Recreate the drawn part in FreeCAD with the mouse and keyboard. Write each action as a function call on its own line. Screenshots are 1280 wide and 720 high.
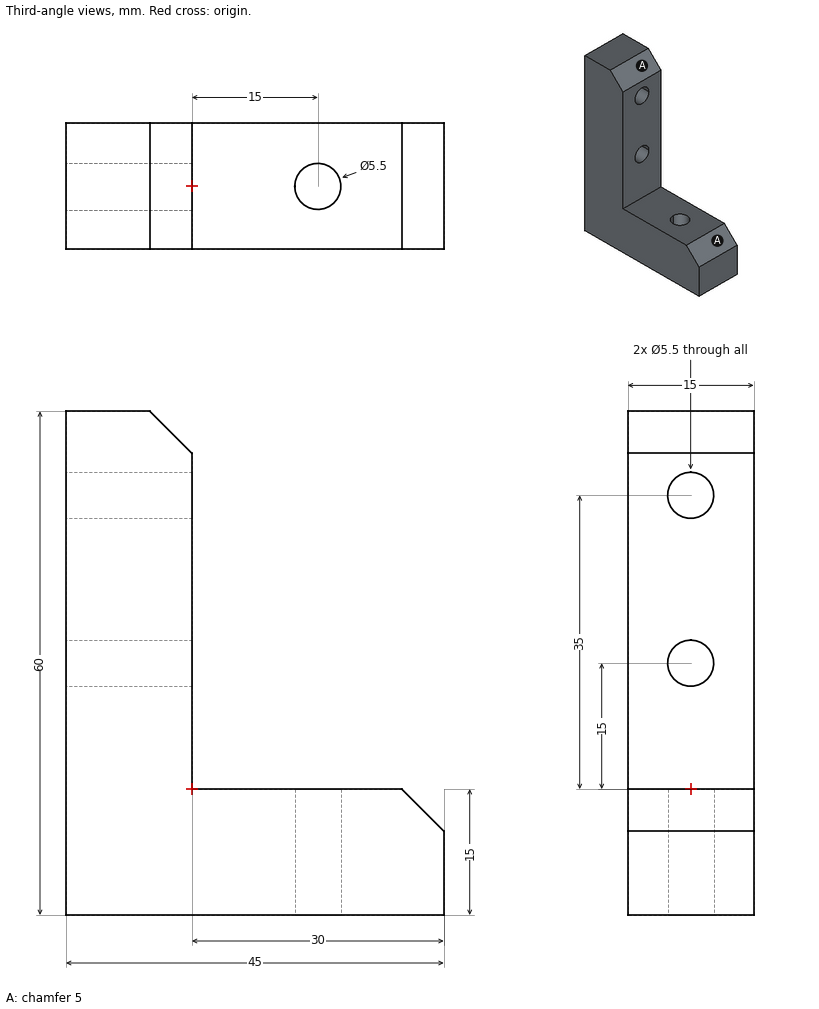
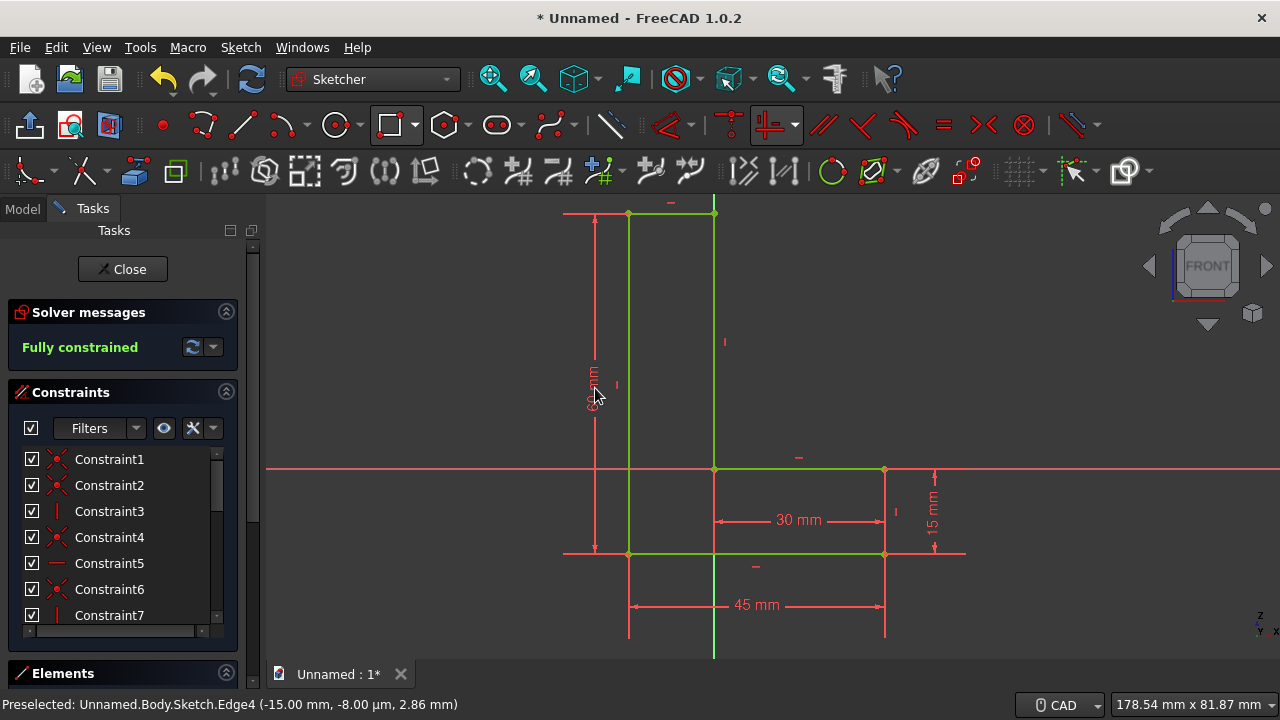
click(123, 269)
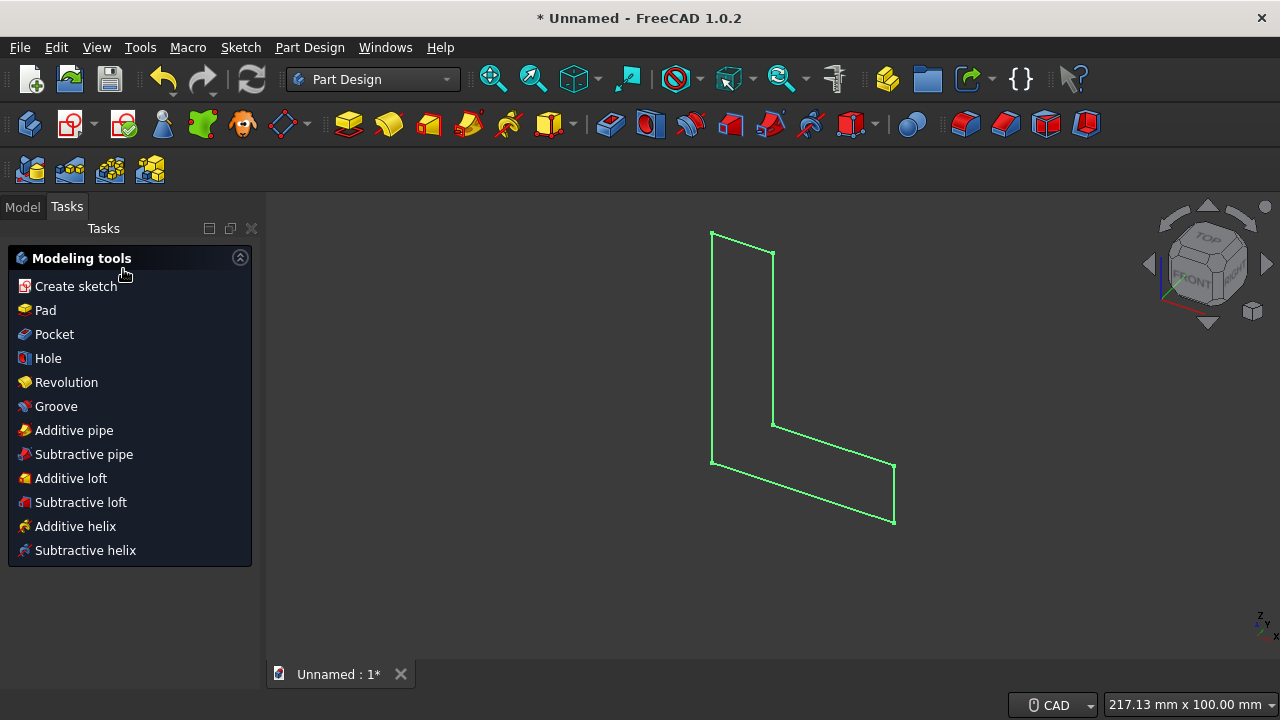
click(350, 124)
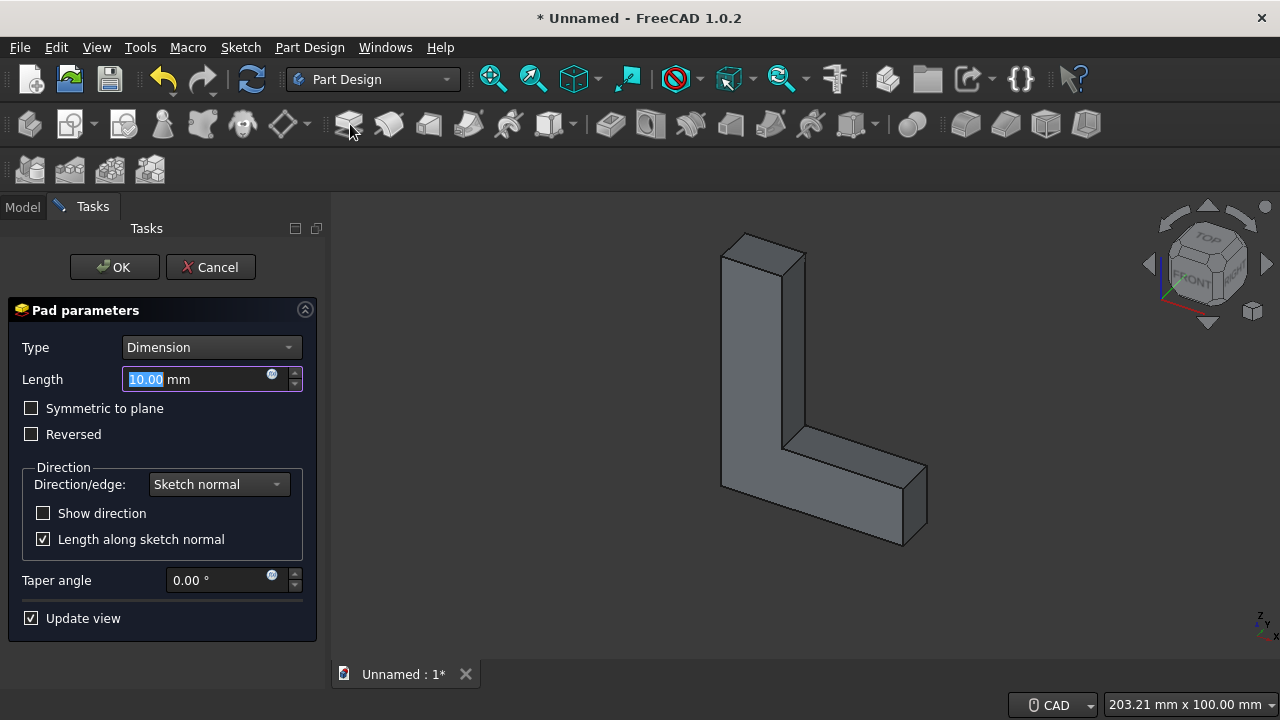
text(15)
key(Tab)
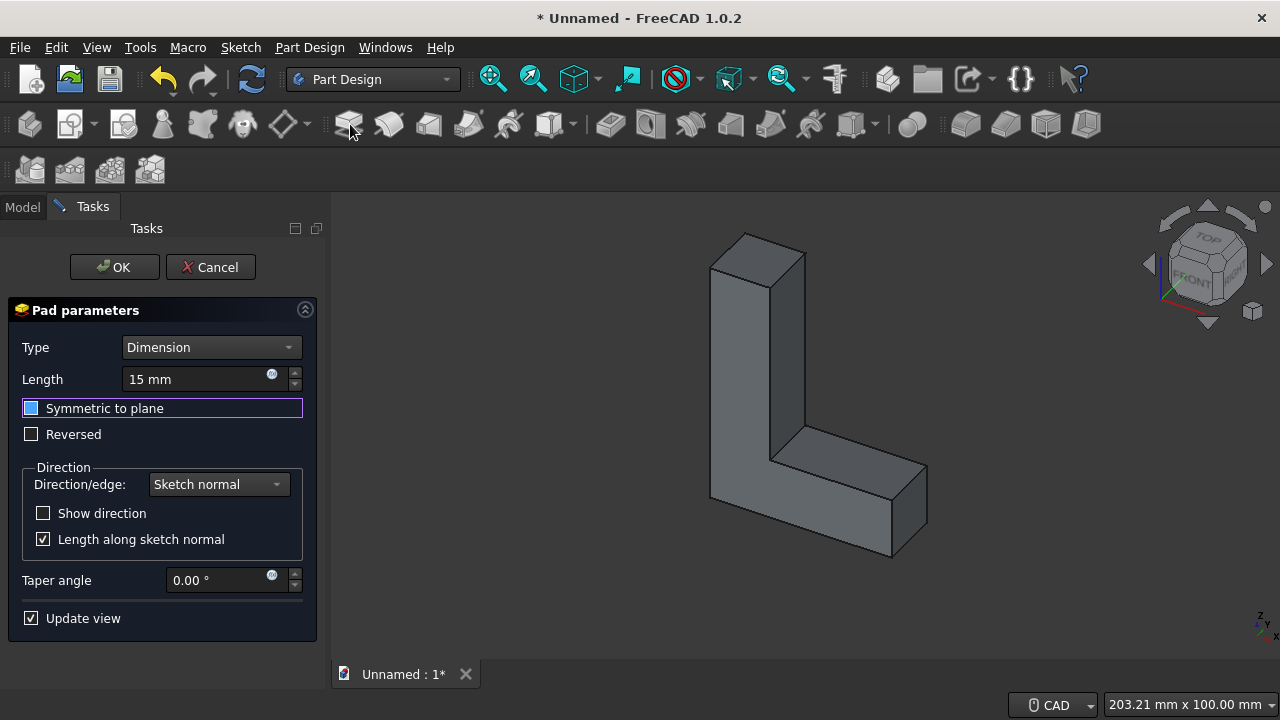
click(30, 408)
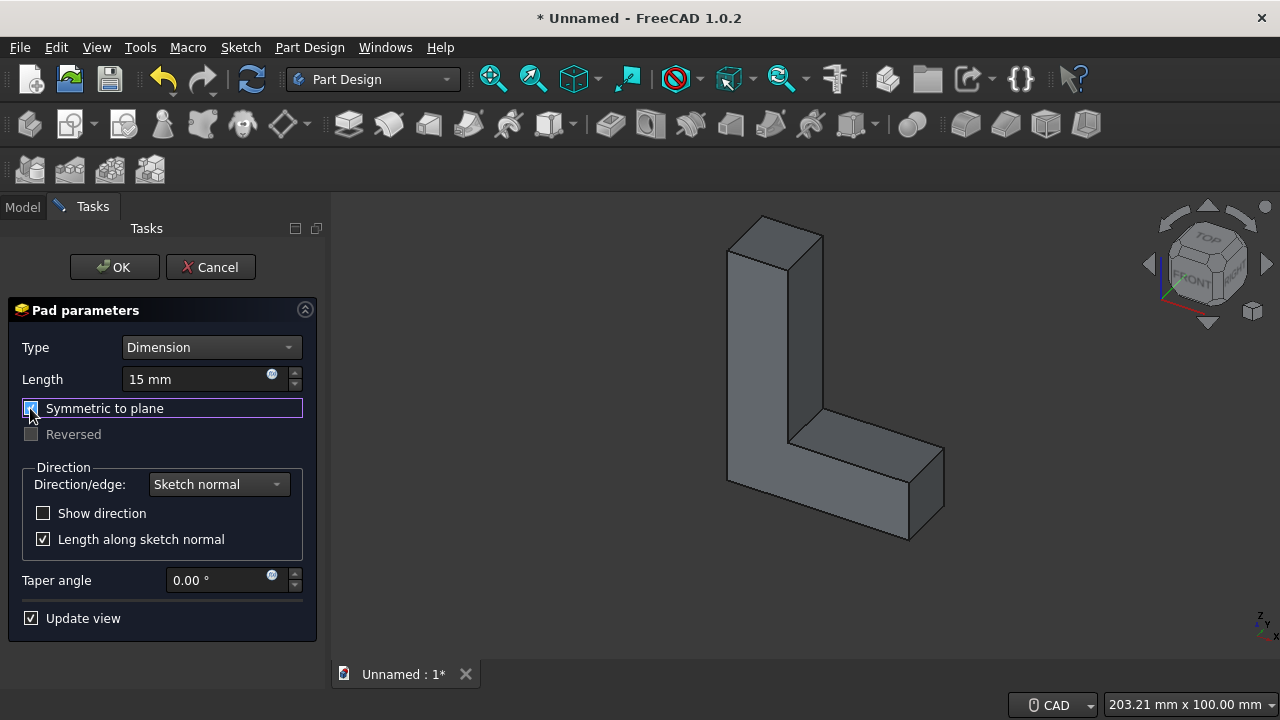
click(115, 267)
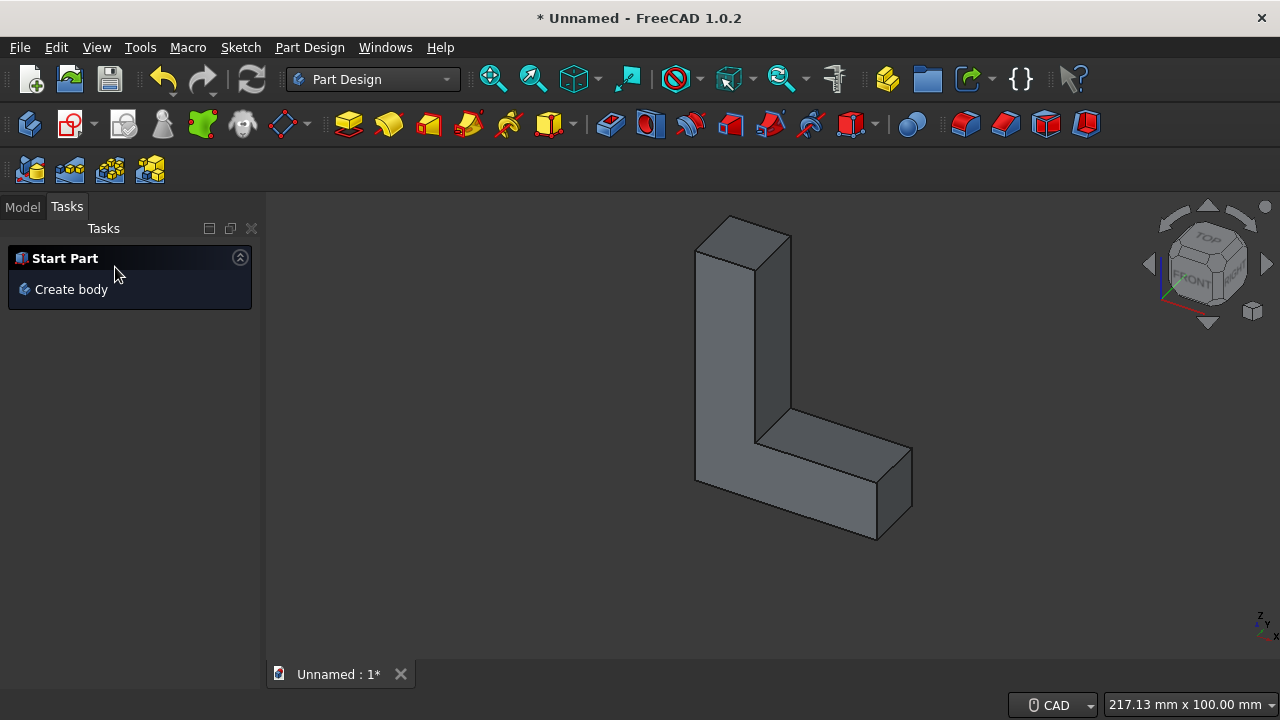
click(894, 465)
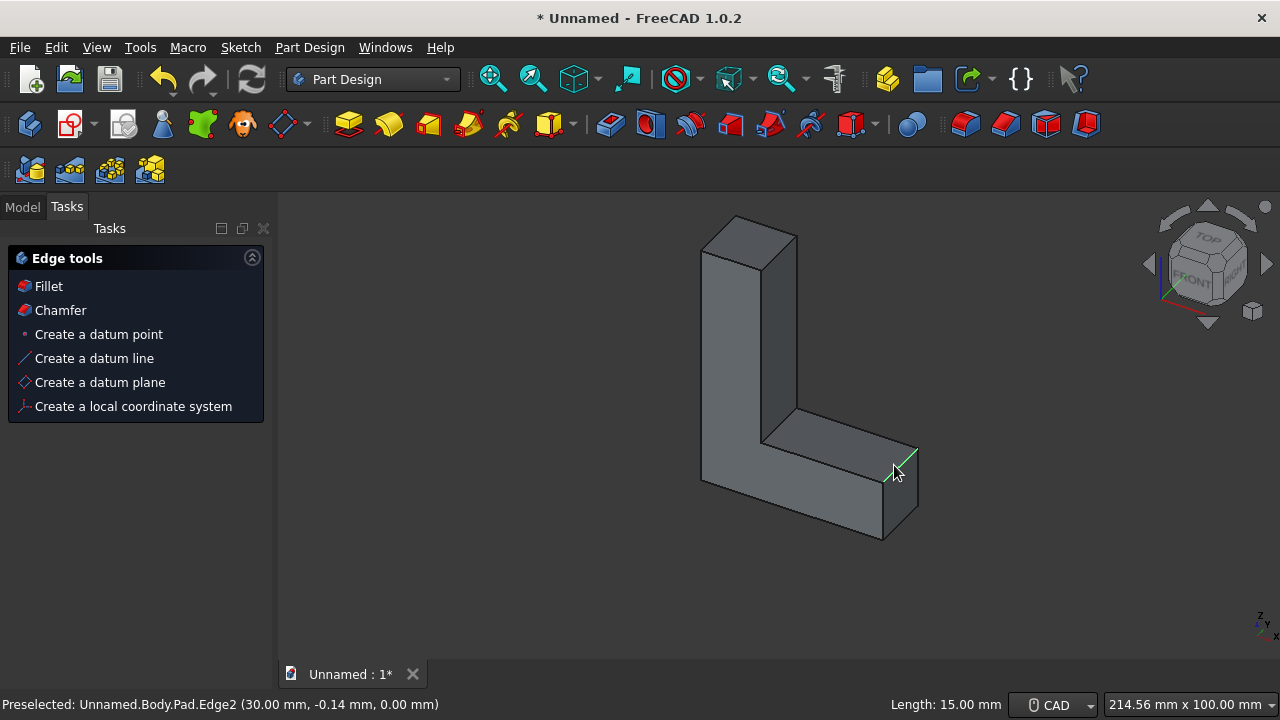
click(779, 252, ctrl)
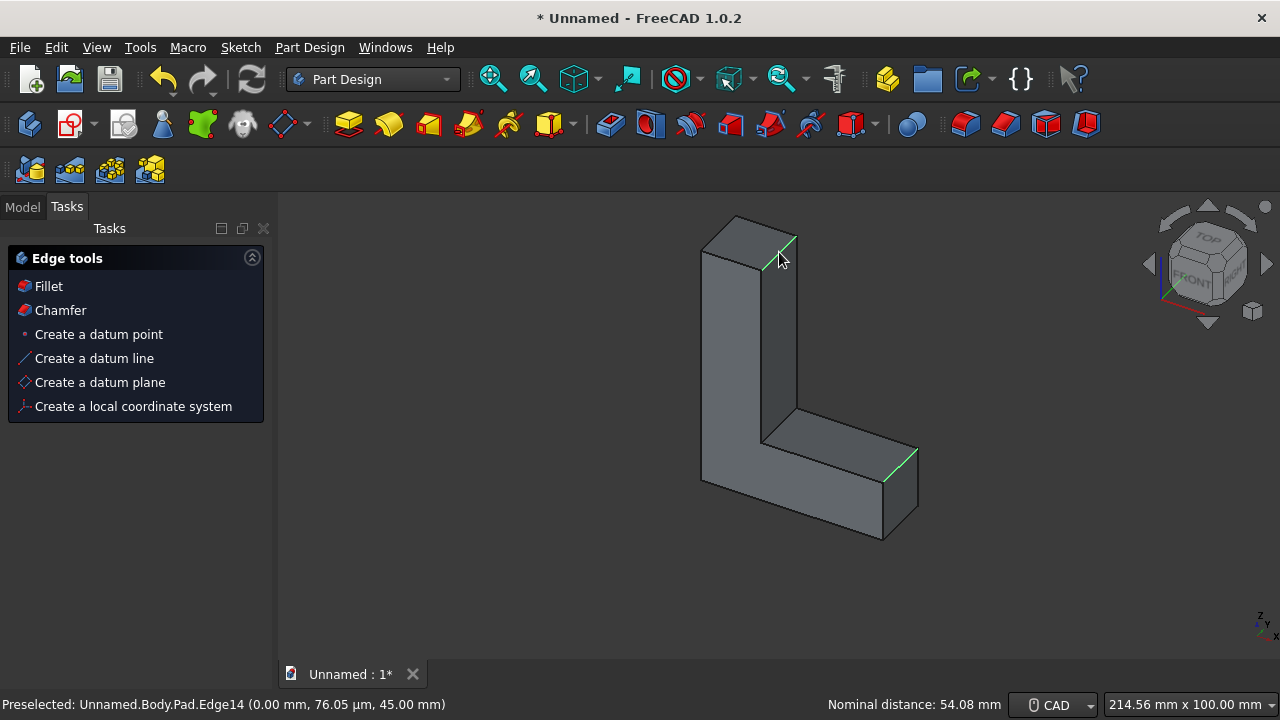
click(1006, 124)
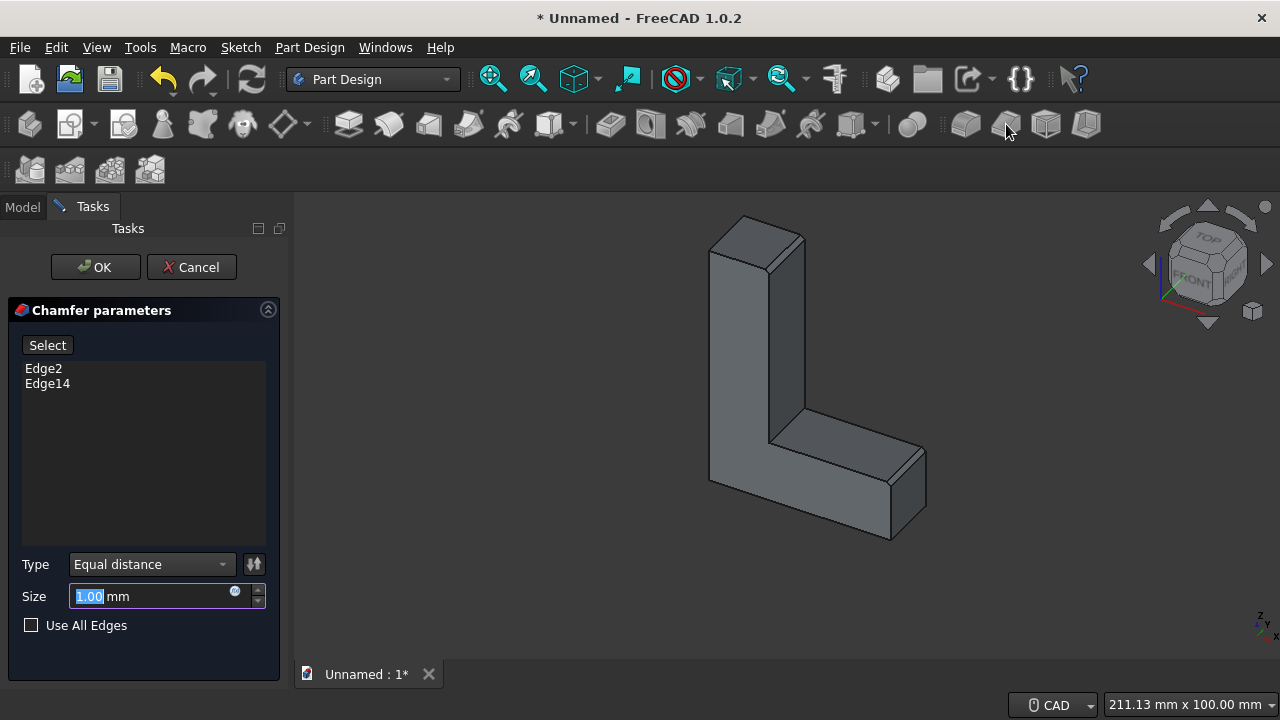
text(5)
key(Tab)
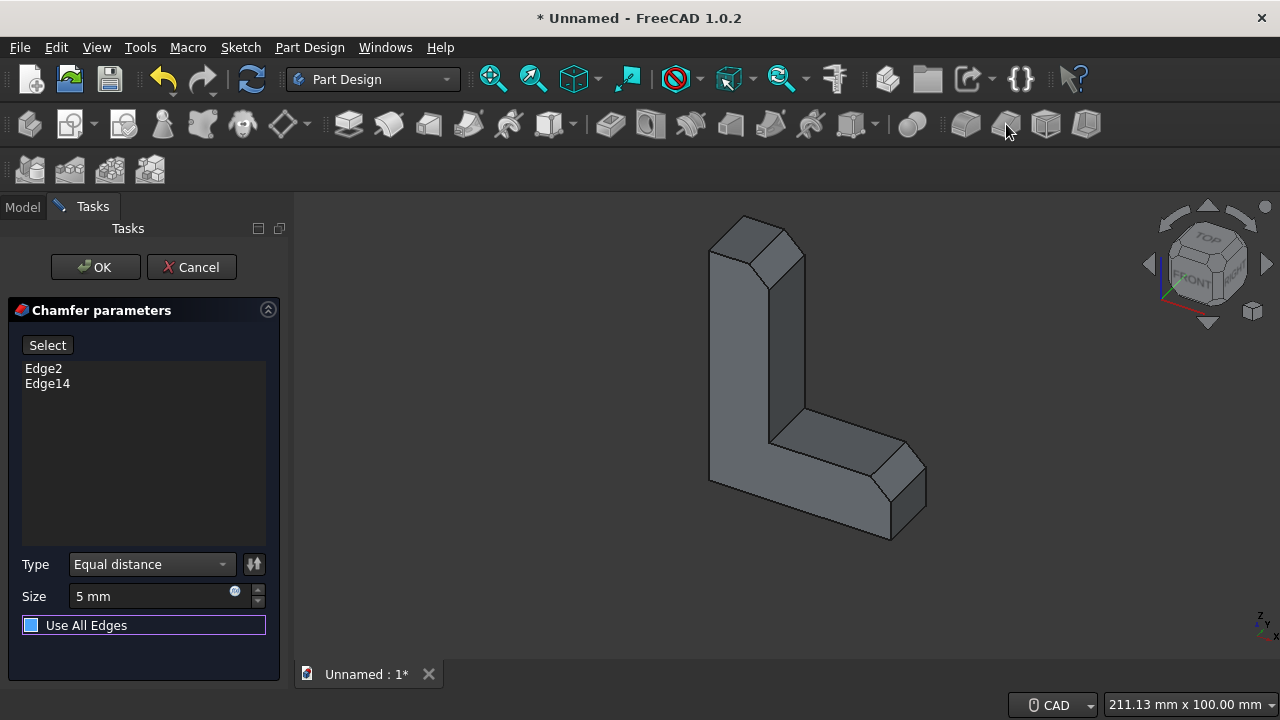
click(96, 267)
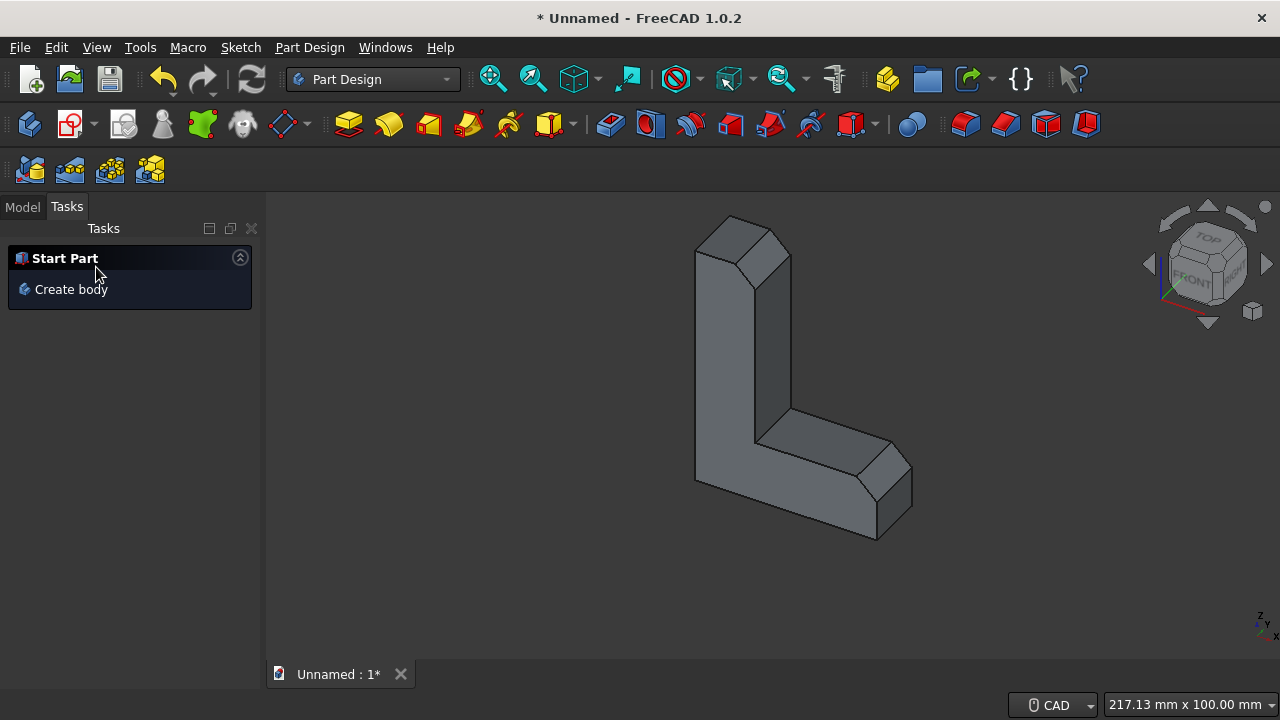
click(70, 124)